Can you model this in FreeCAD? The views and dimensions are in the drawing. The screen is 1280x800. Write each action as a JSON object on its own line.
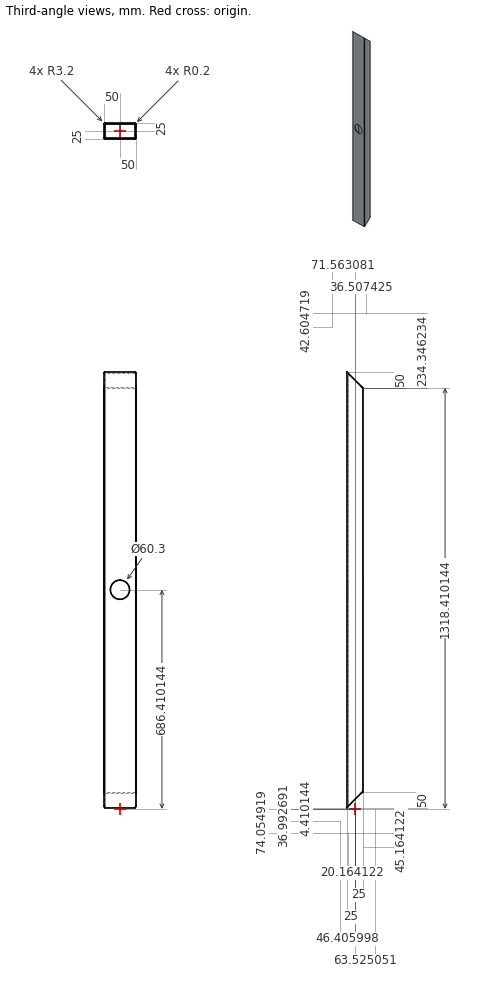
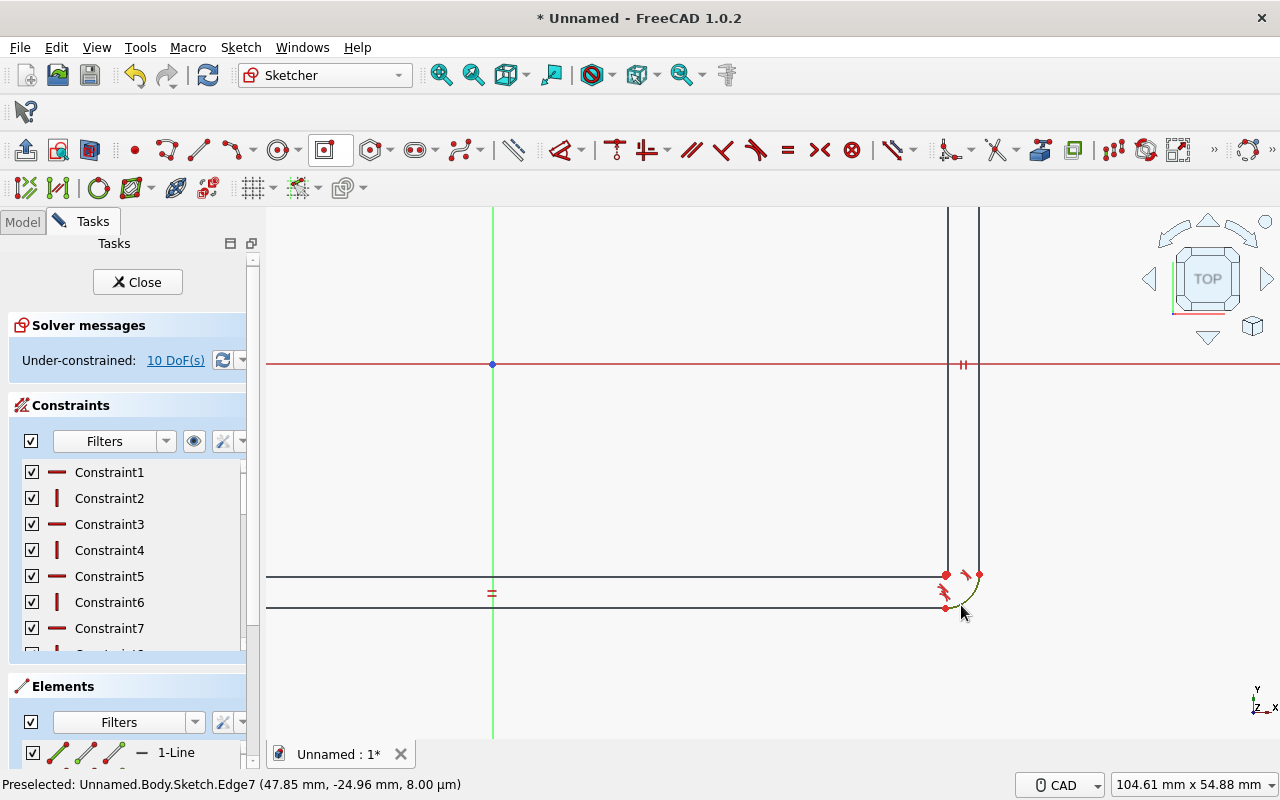
{"action": "scroll", "coordinate": [962, 605], "scroll_direction": "down", "scroll_amount": 3}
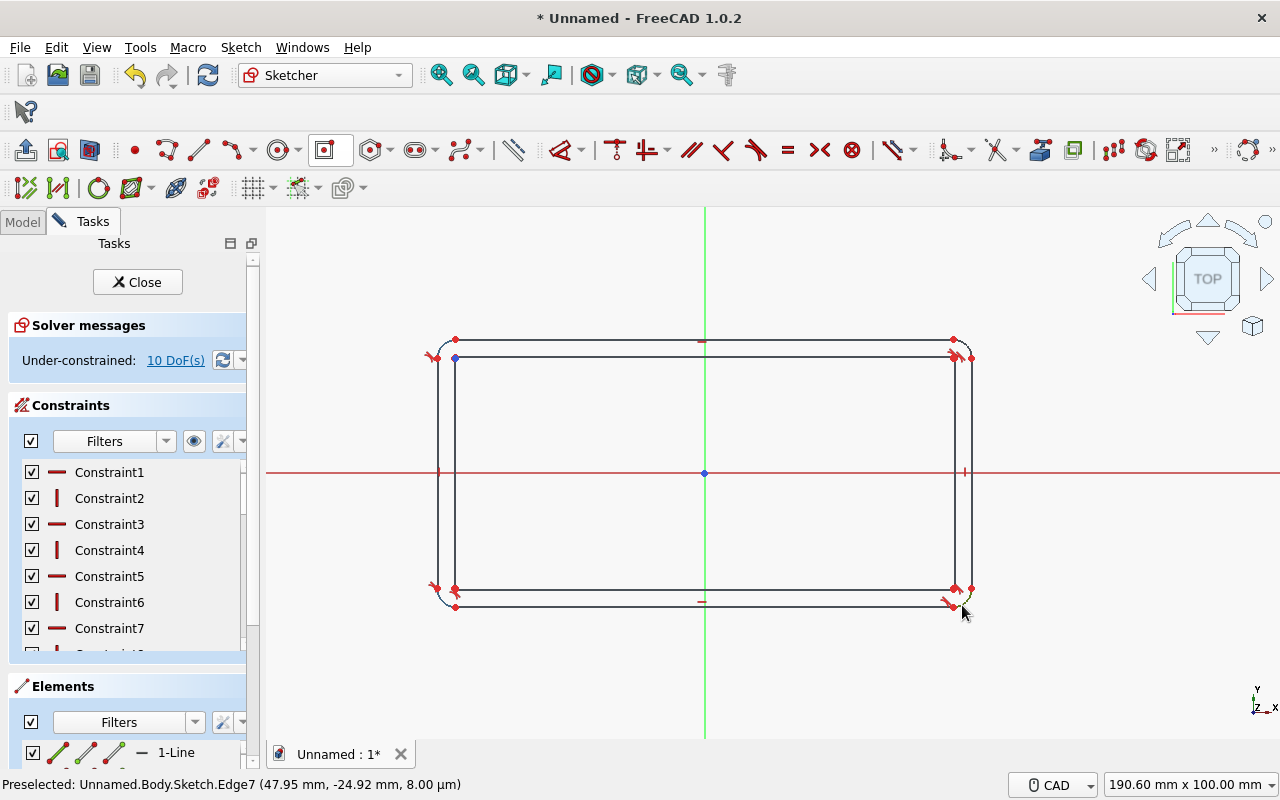
{"action": "scroll", "coordinate": [970, 350], "scroll_direction": "up", "scroll_amount": 3}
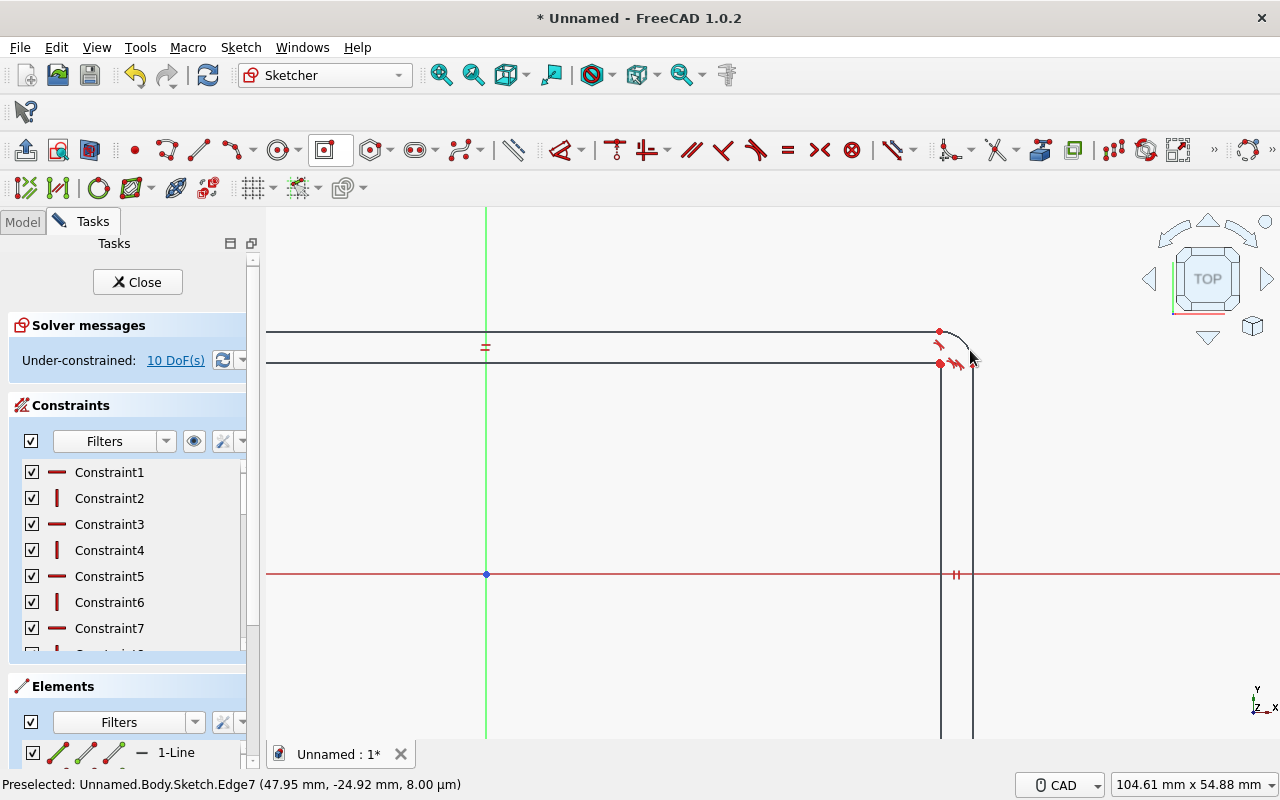
{"action": "left_click", "coordinate": [969, 350]}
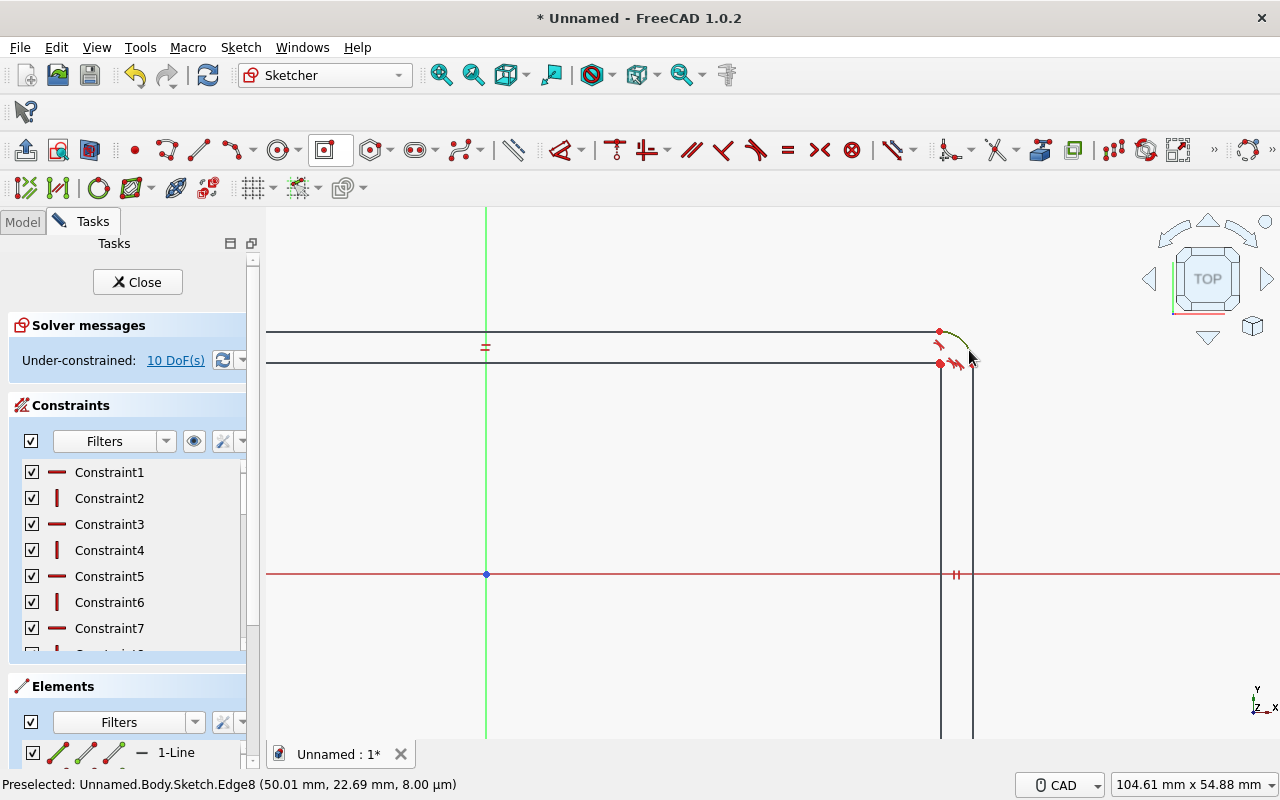
{"action": "left_click", "coordinate": [788, 150]}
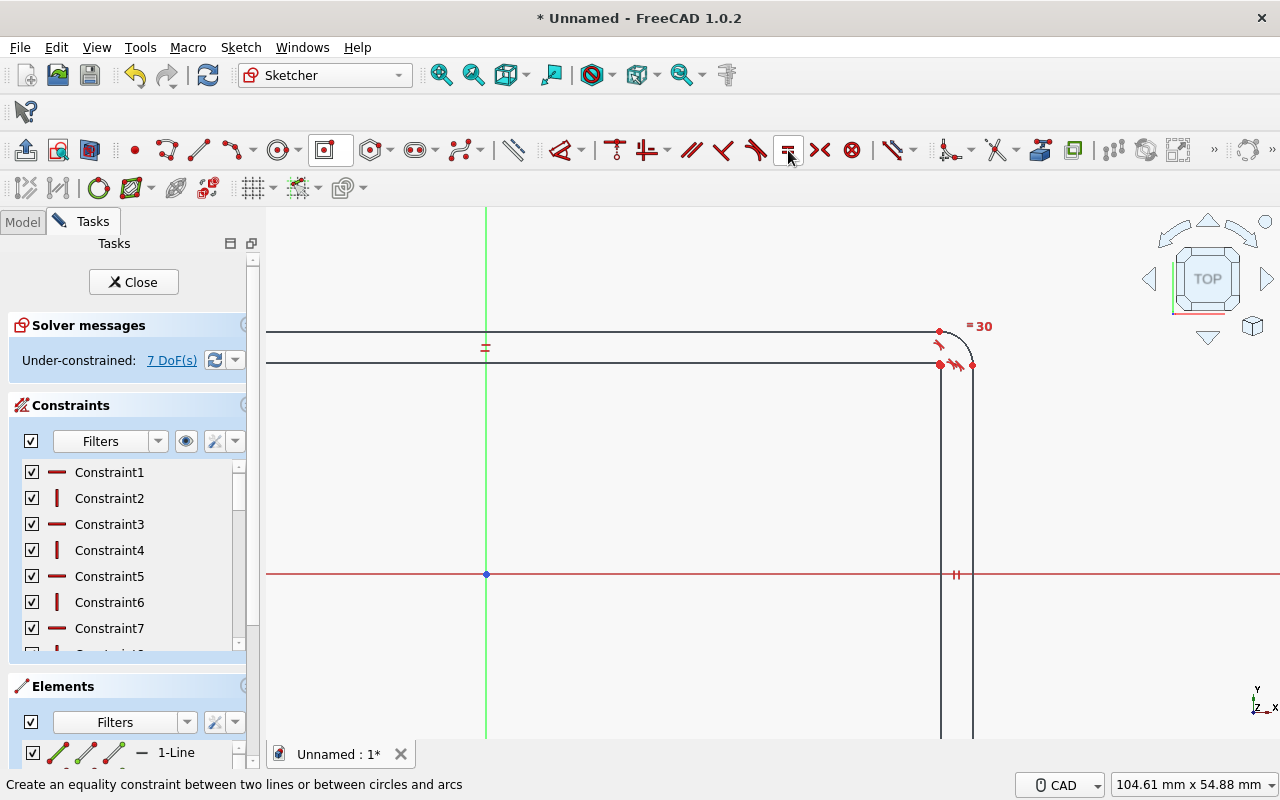
{"action": "scroll", "coordinate": [940, 364], "scroll_direction": "up", "scroll_amount": 11}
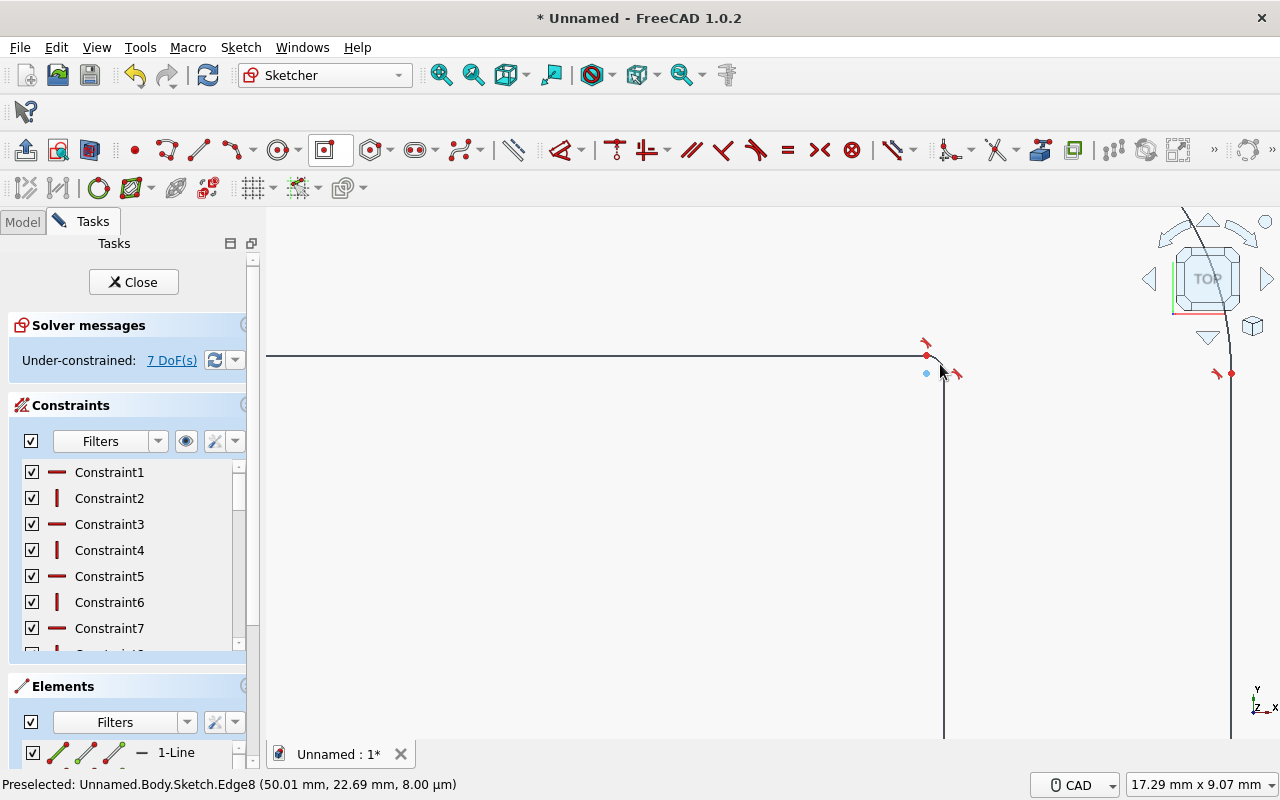
{"action": "left_click", "coordinate": [939, 361]}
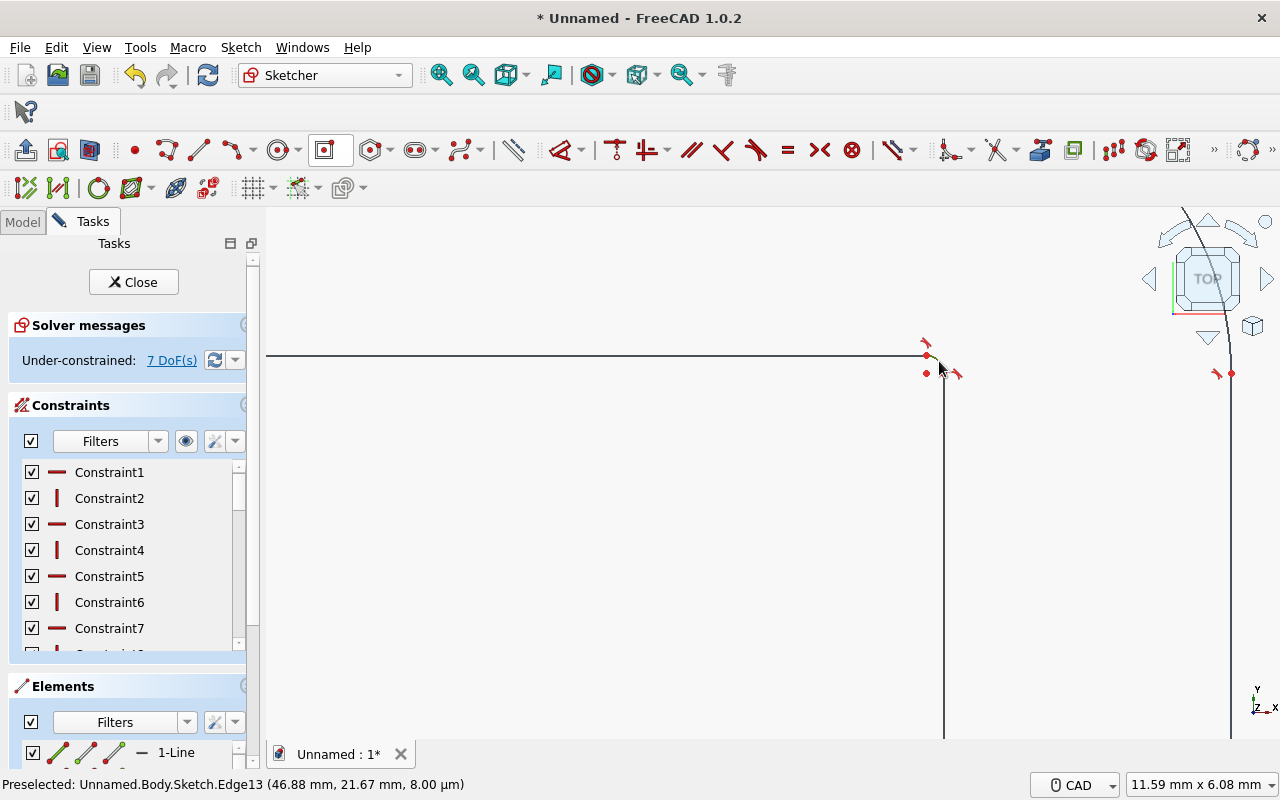
{"action": "scroll", "coordinate": [955, 357], "scroll_direction": "down", "scroll_amount": 14}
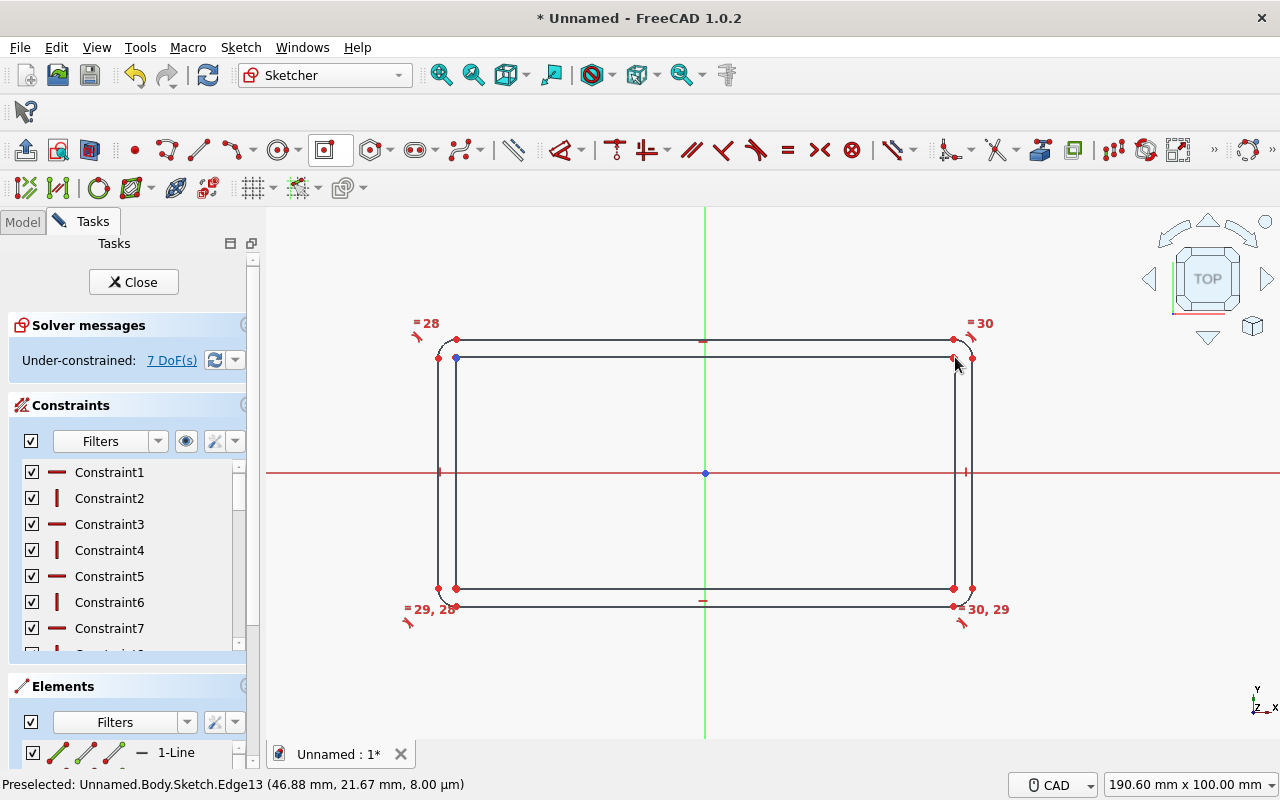
{"action": "scroll", "coordinate": [456, 357], "scroll_direction": "up", "scroll_amount": 14}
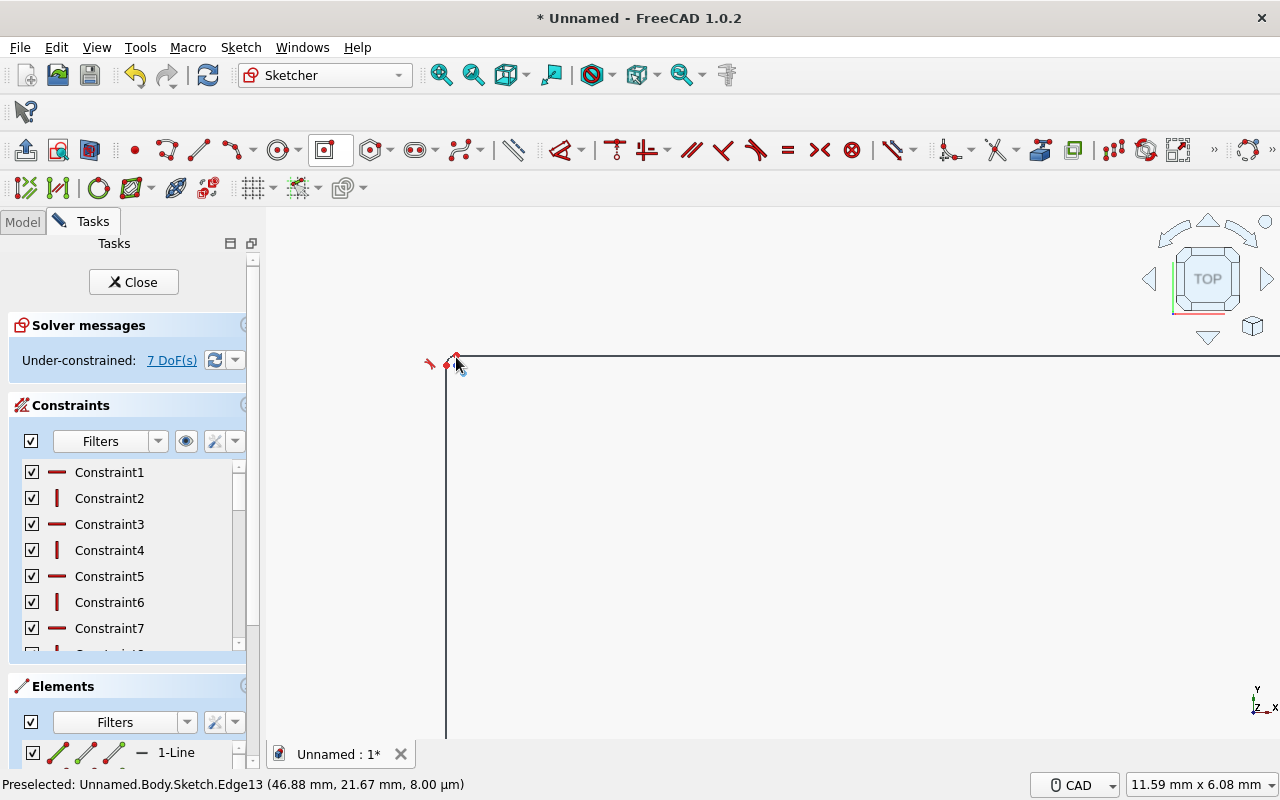
{"action": "left_click", "coordinate": [449, 359]}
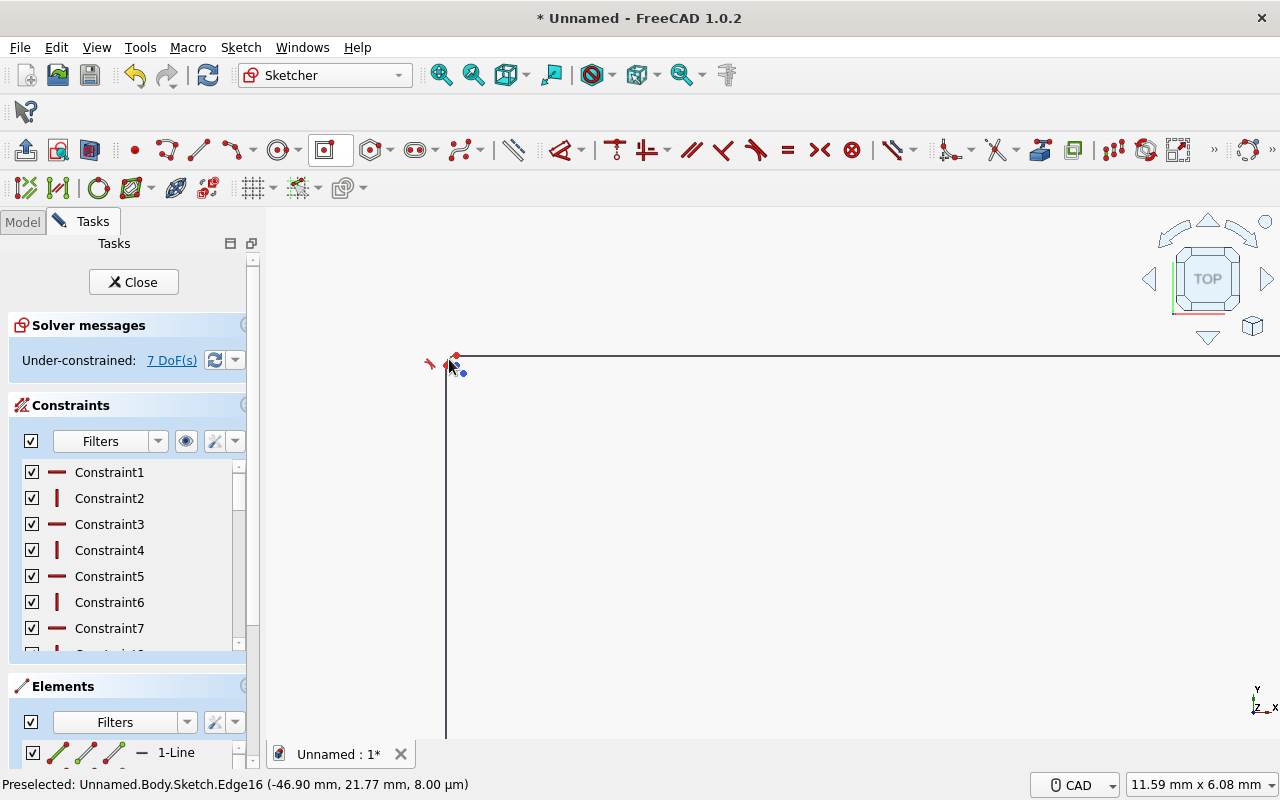
{"action": "left_click", "coordinate": [788, 150]}